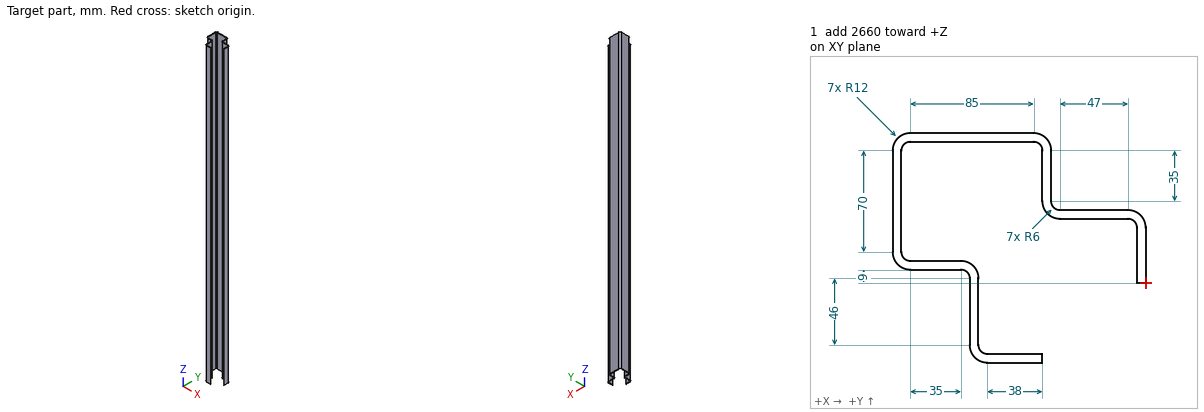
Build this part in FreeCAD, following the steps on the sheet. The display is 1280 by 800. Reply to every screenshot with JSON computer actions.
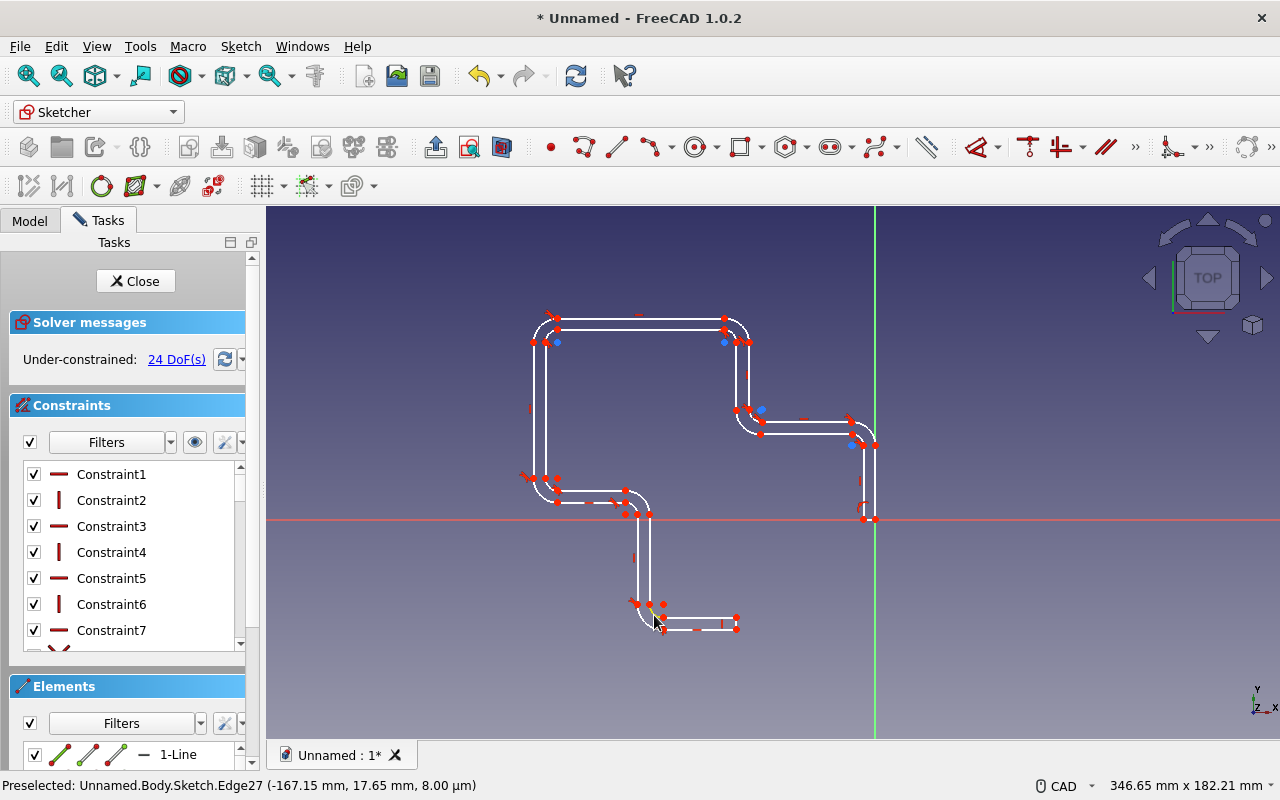
{"action": "scroll", "coordinate": [547, 321], "scroll_direction": "up", "scroll_amount": 2}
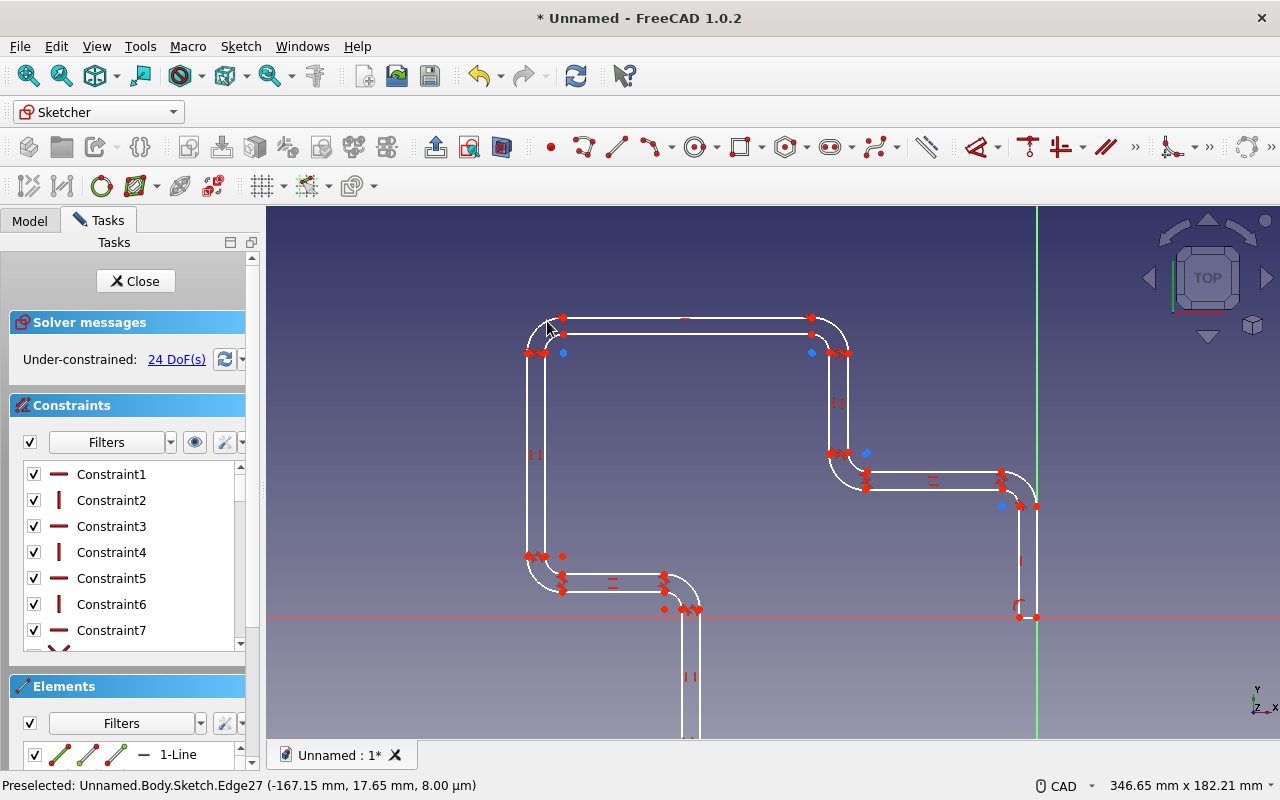
{"action": "left_click", "coordinate": [547, 322]}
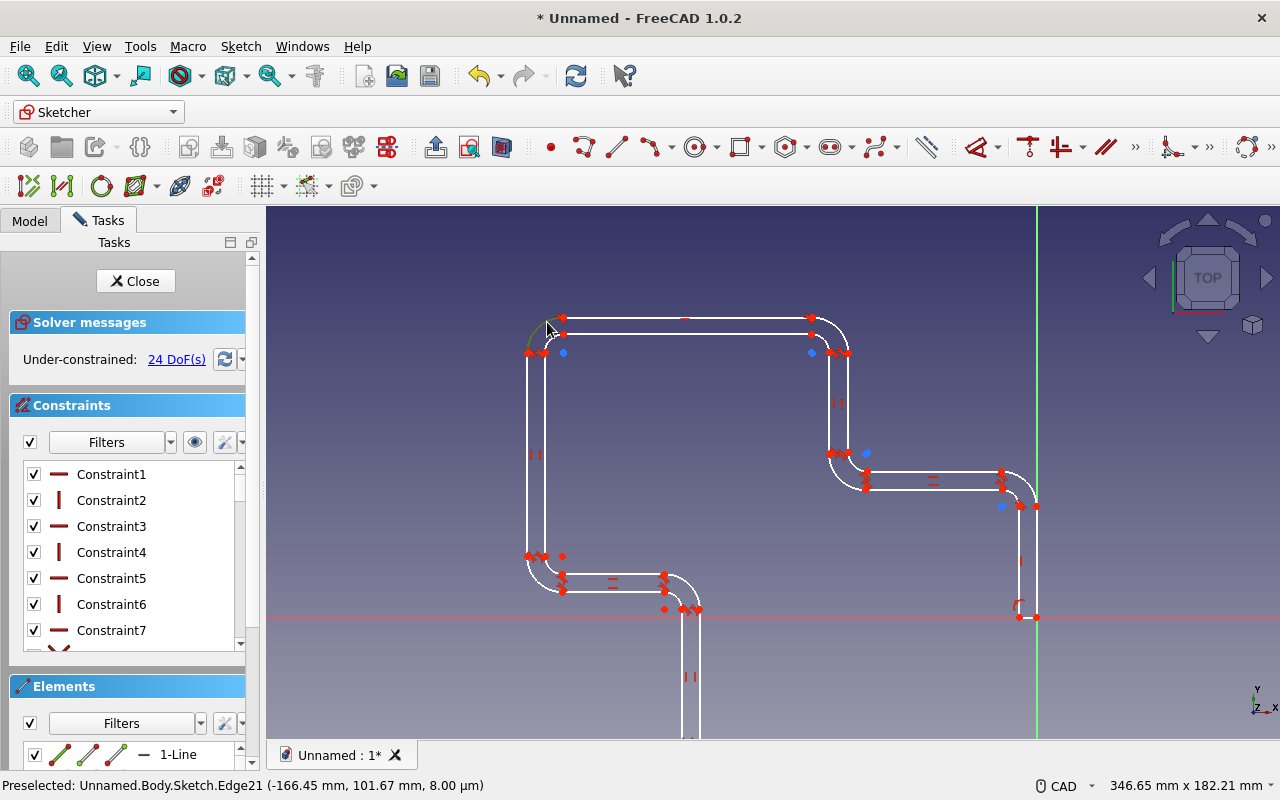
{"action": "left_click", "coordinate": [550, 340]}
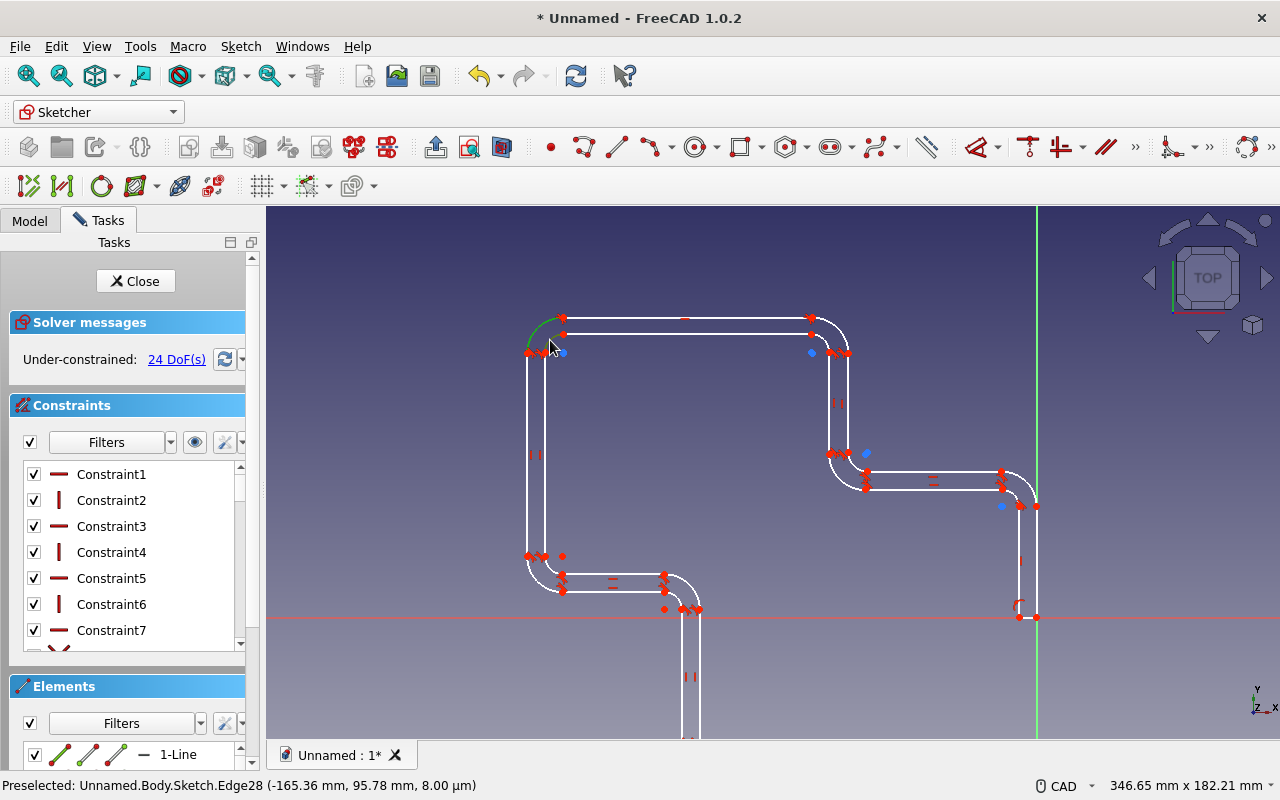
{"action": "key", "text": "c"}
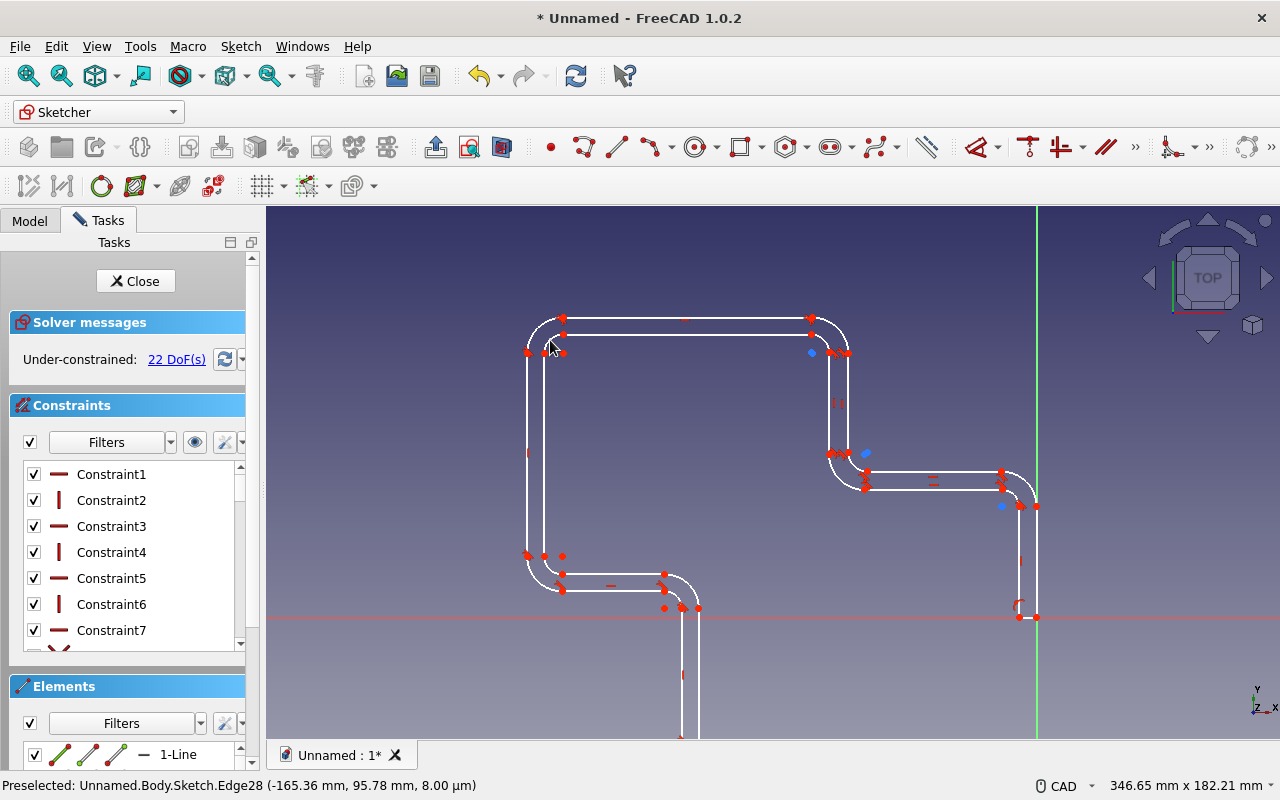
{"action": "left_click", "coordinate": [844, 337]}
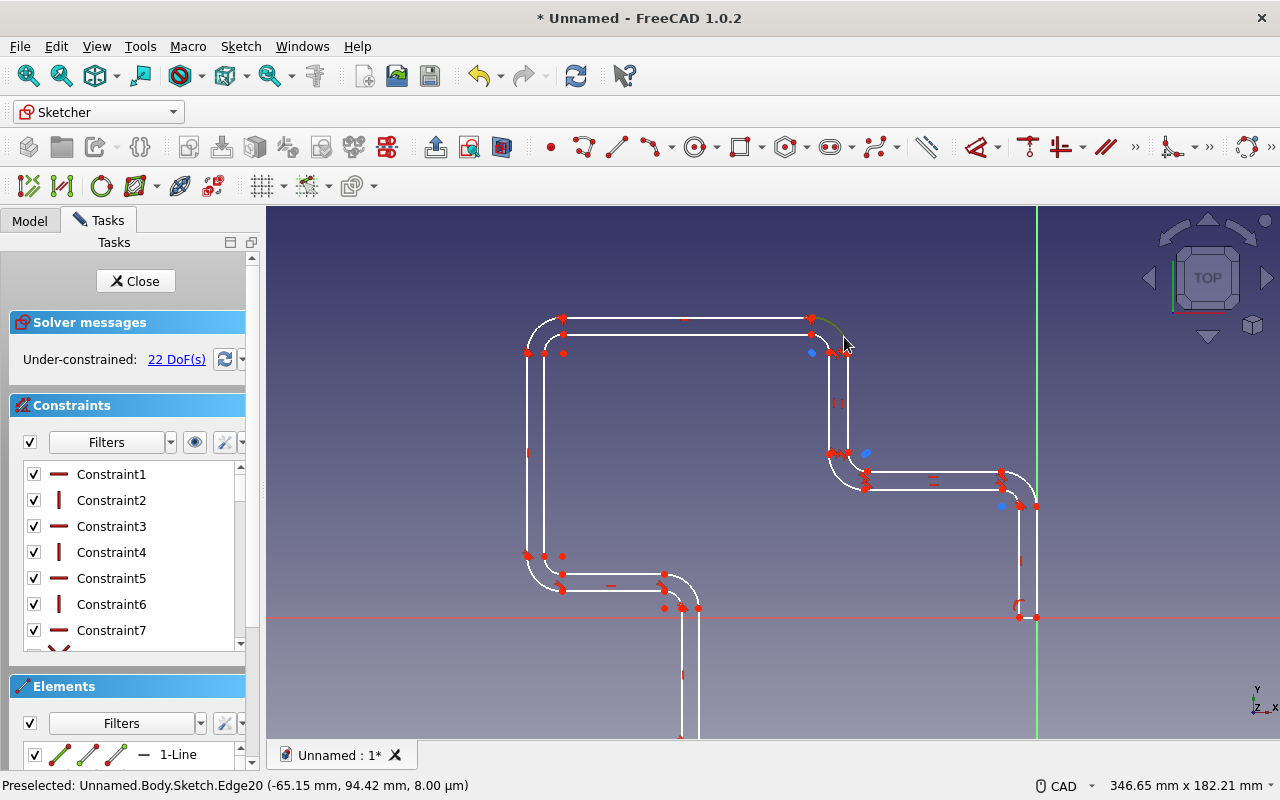
{"action": "left_click", "coordinate": [824, 340]}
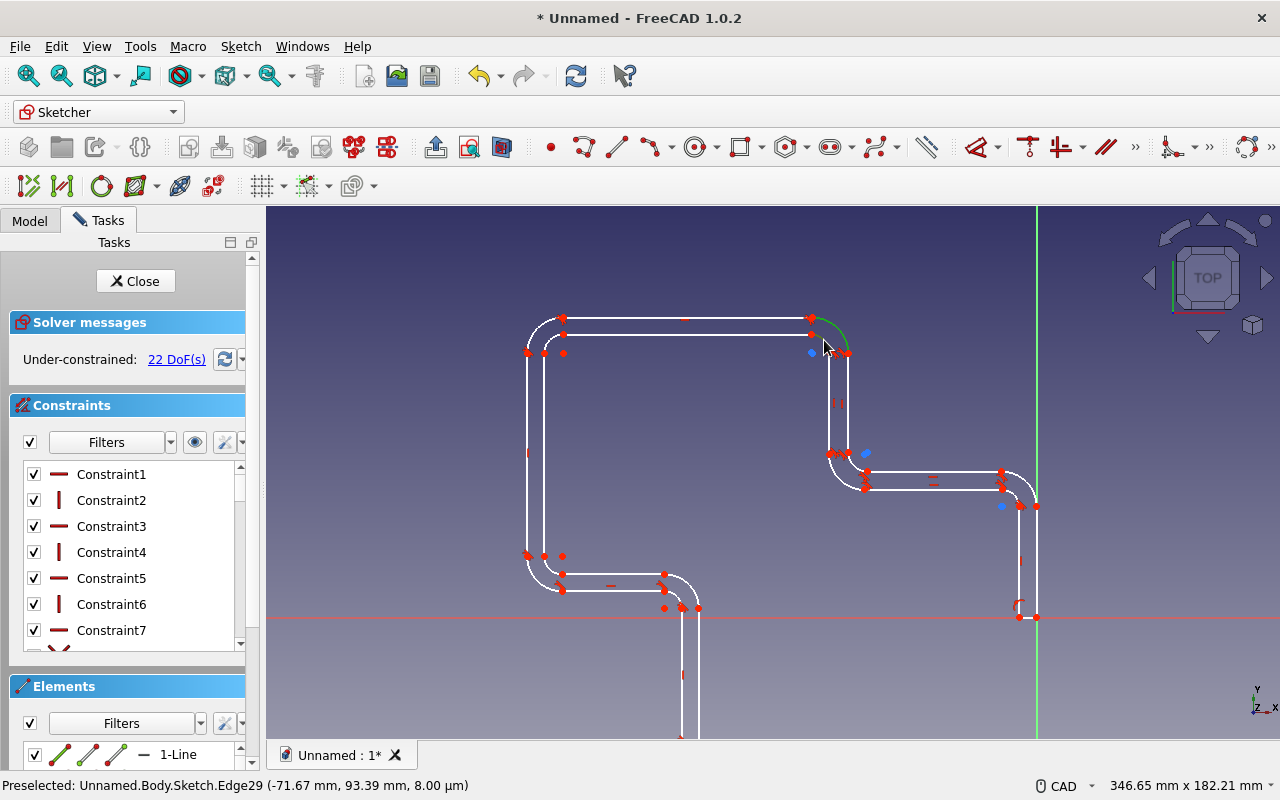
{"action": "key", "text": "c"}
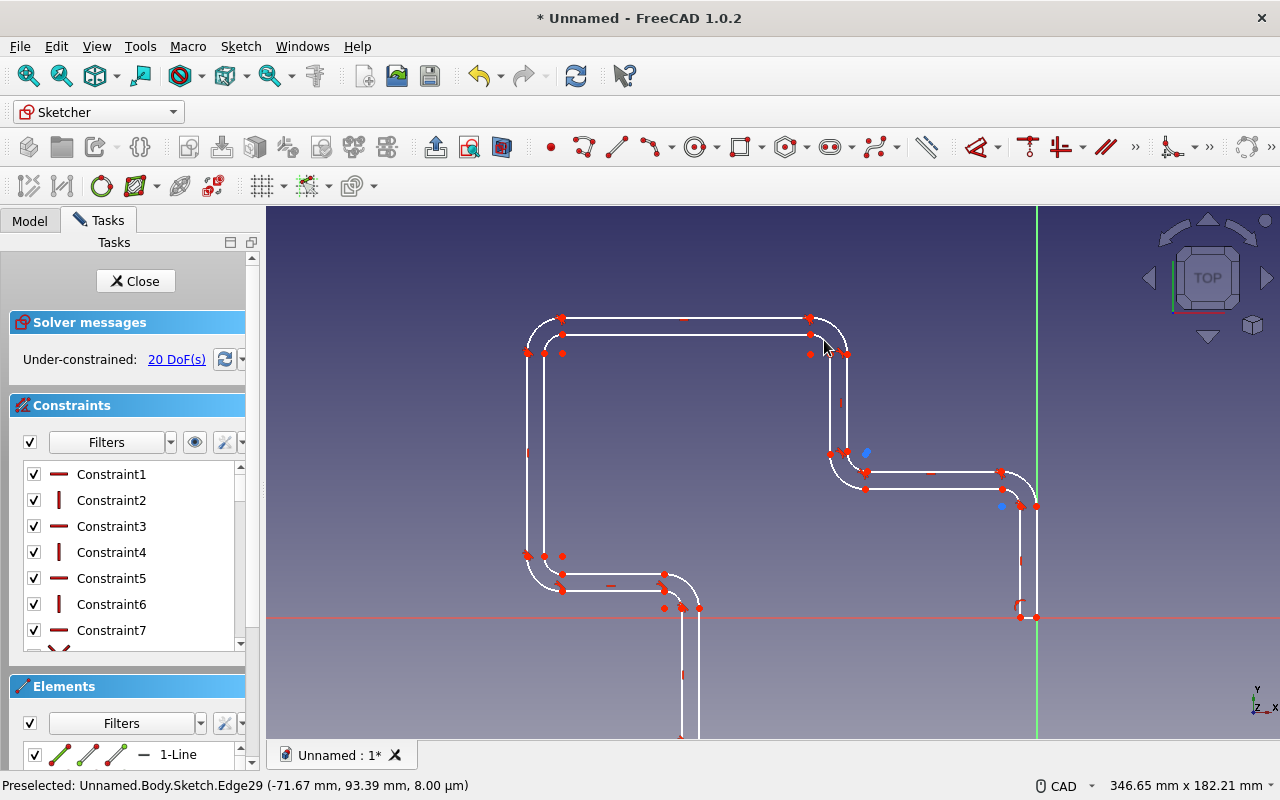
{"action": "scroll", "coordinate": [849, 460], "scroll_direction": "up", "scroll_amount": 2}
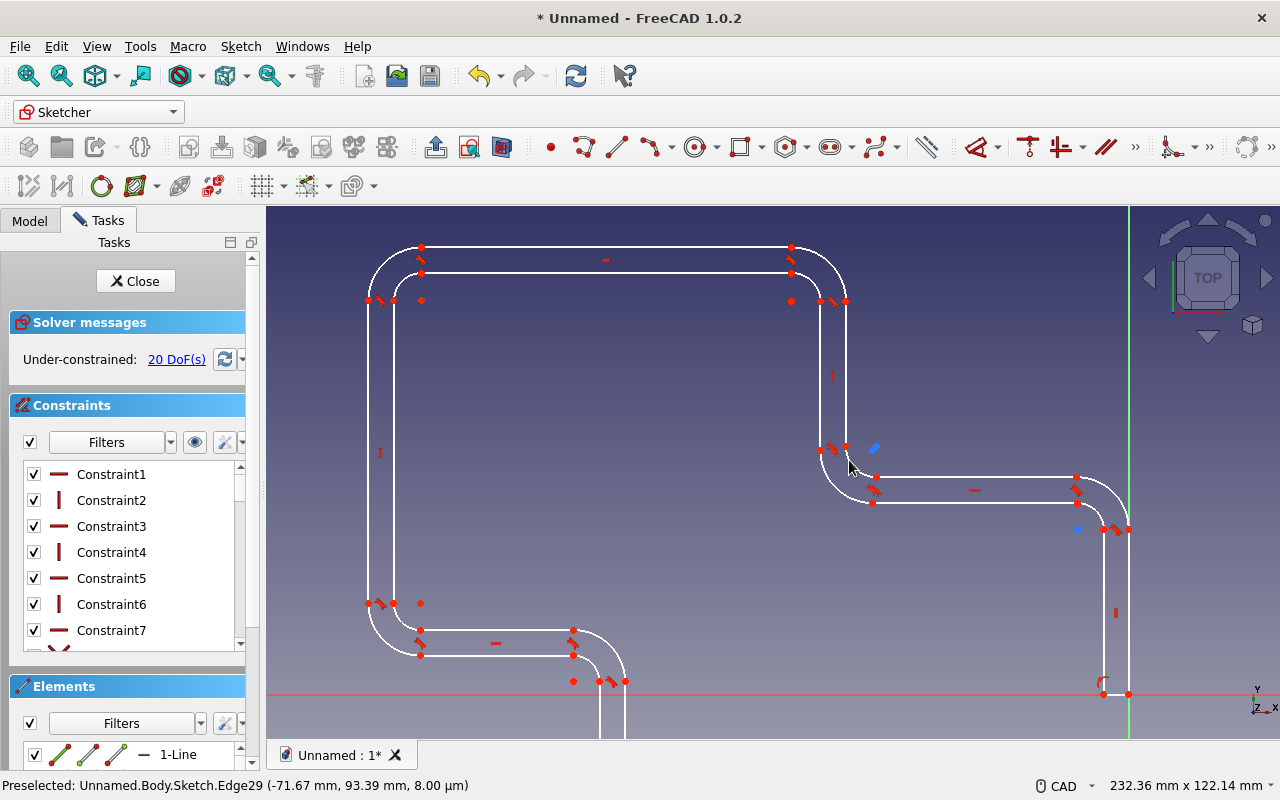
{"action": "left_click", "coordinate": [849, 460]}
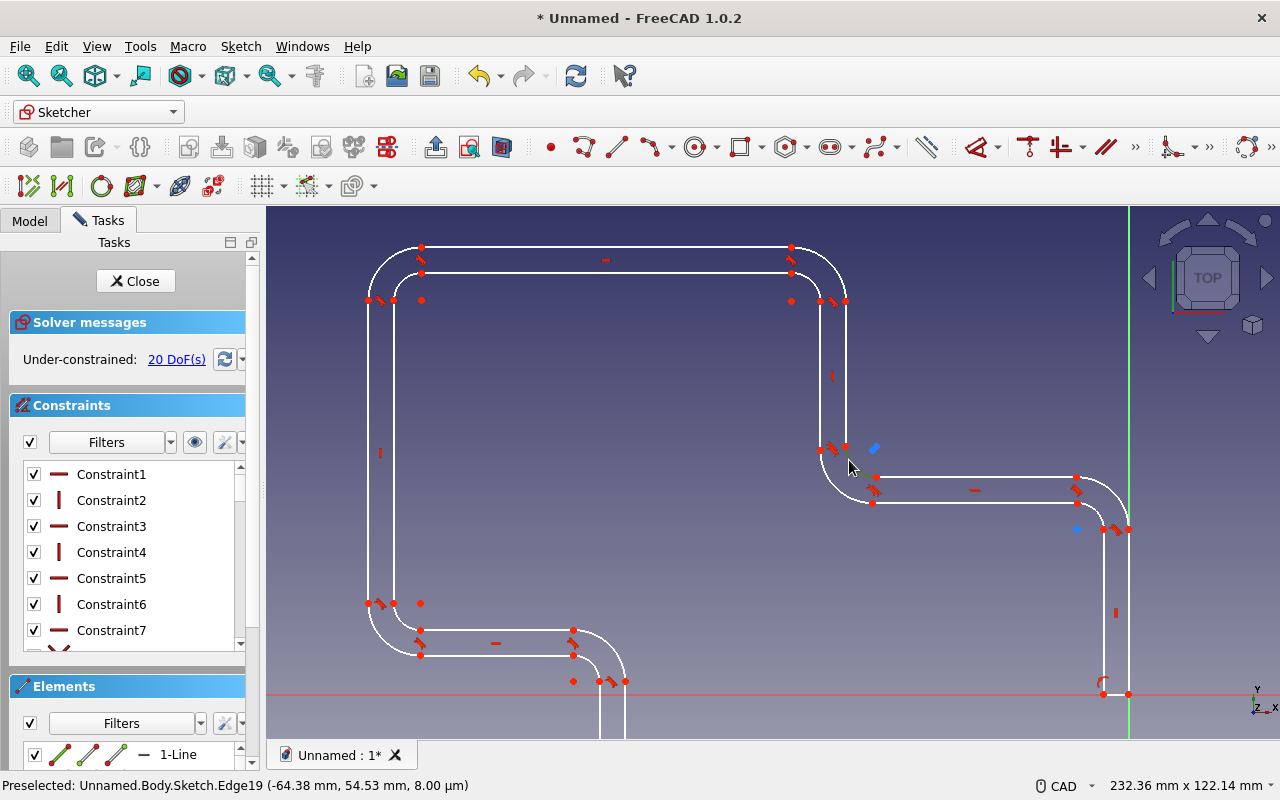
{"action": "left_click", "coordinate": [826, 475]}